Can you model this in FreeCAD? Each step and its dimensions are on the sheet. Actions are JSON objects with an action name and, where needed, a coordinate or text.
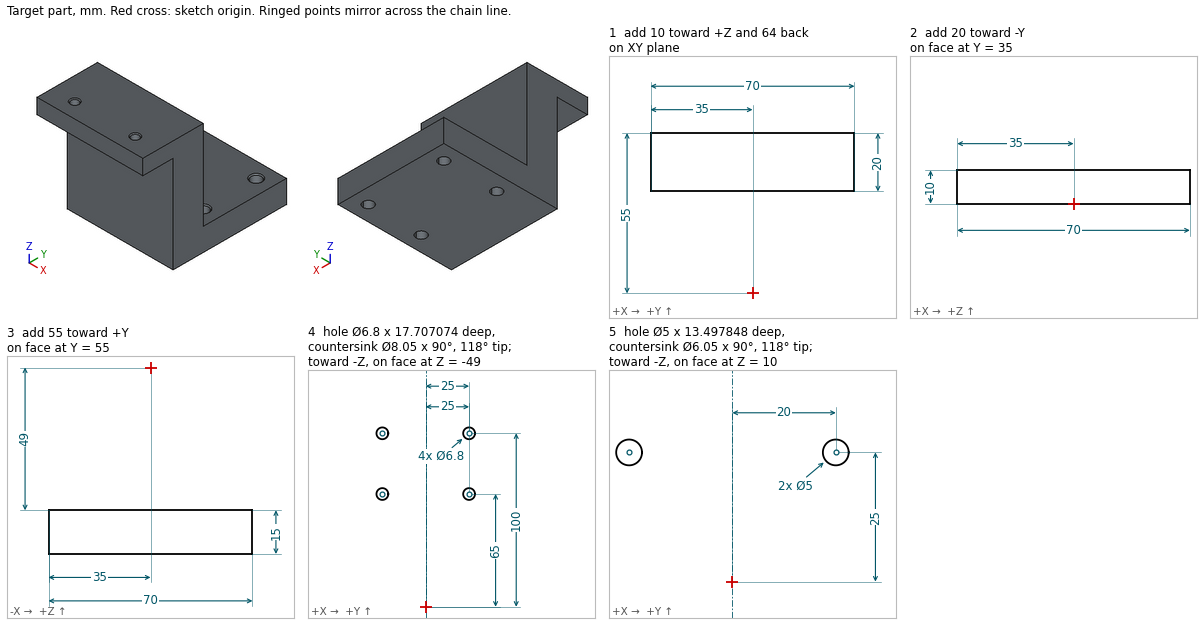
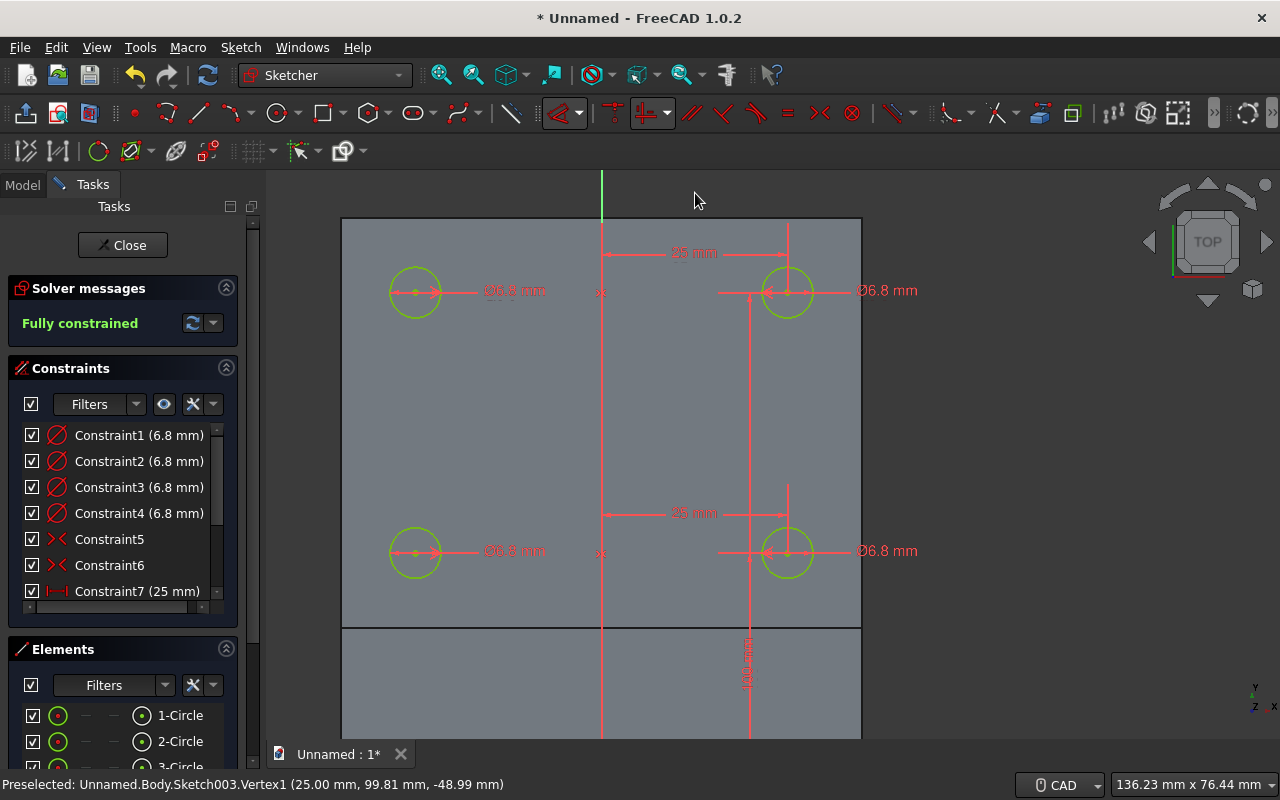
{"action": "left_click", "coordinate": [123, 245]}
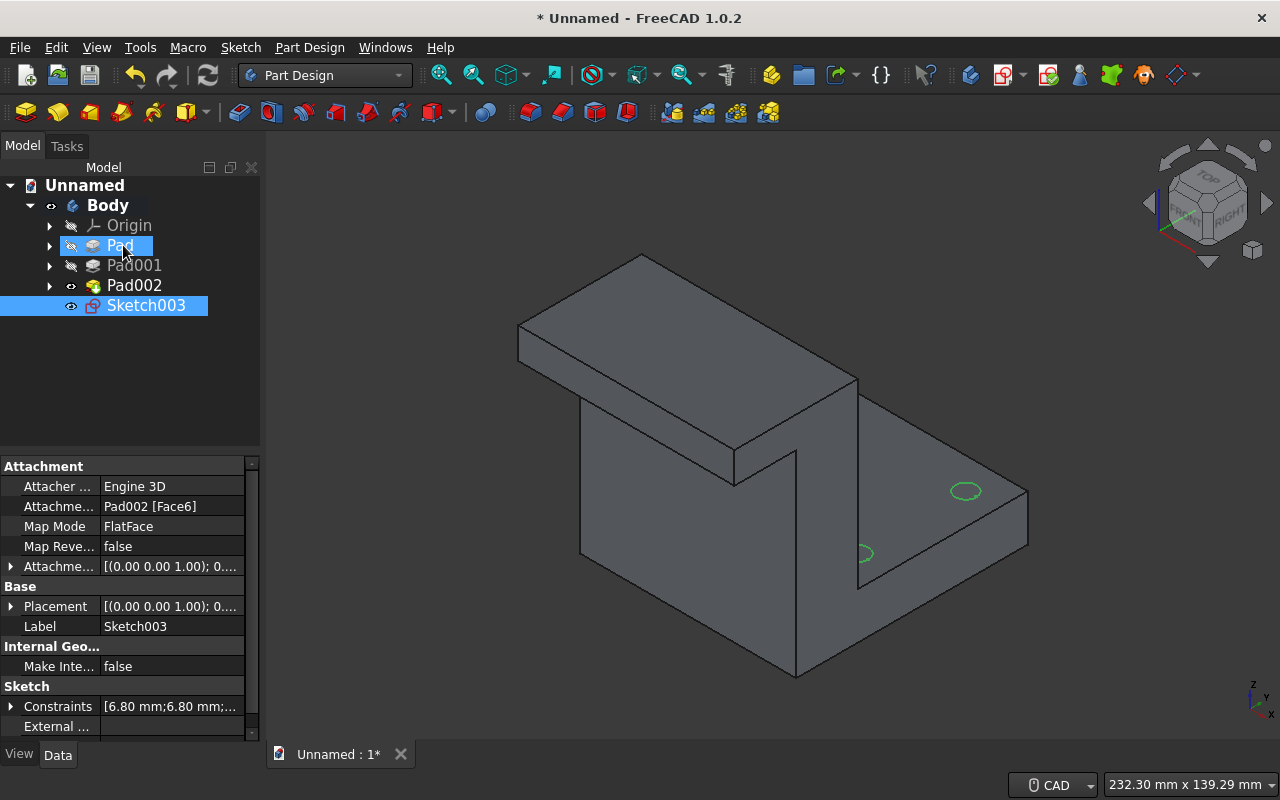
{"action": "left_click", "coordinate": [272, 112]}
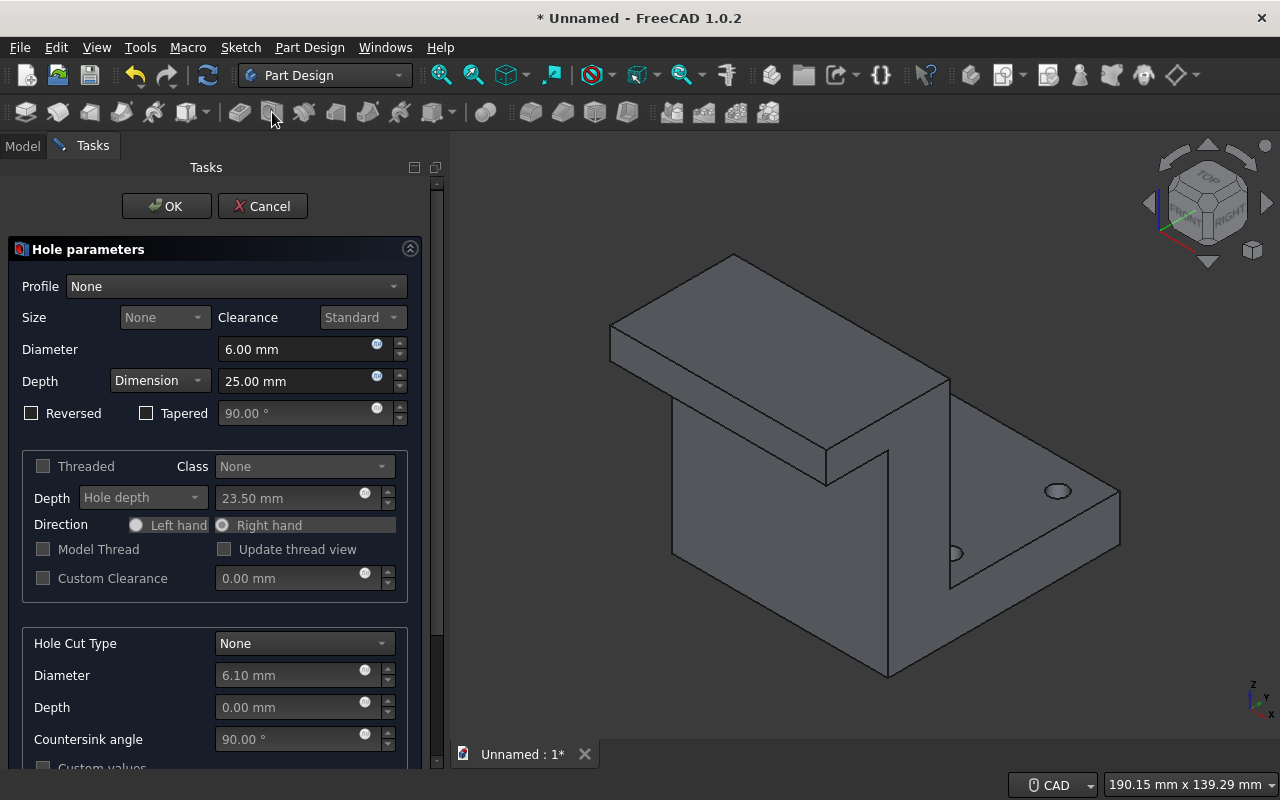
{"action": "triple_click", "coordinate": [305, 349]}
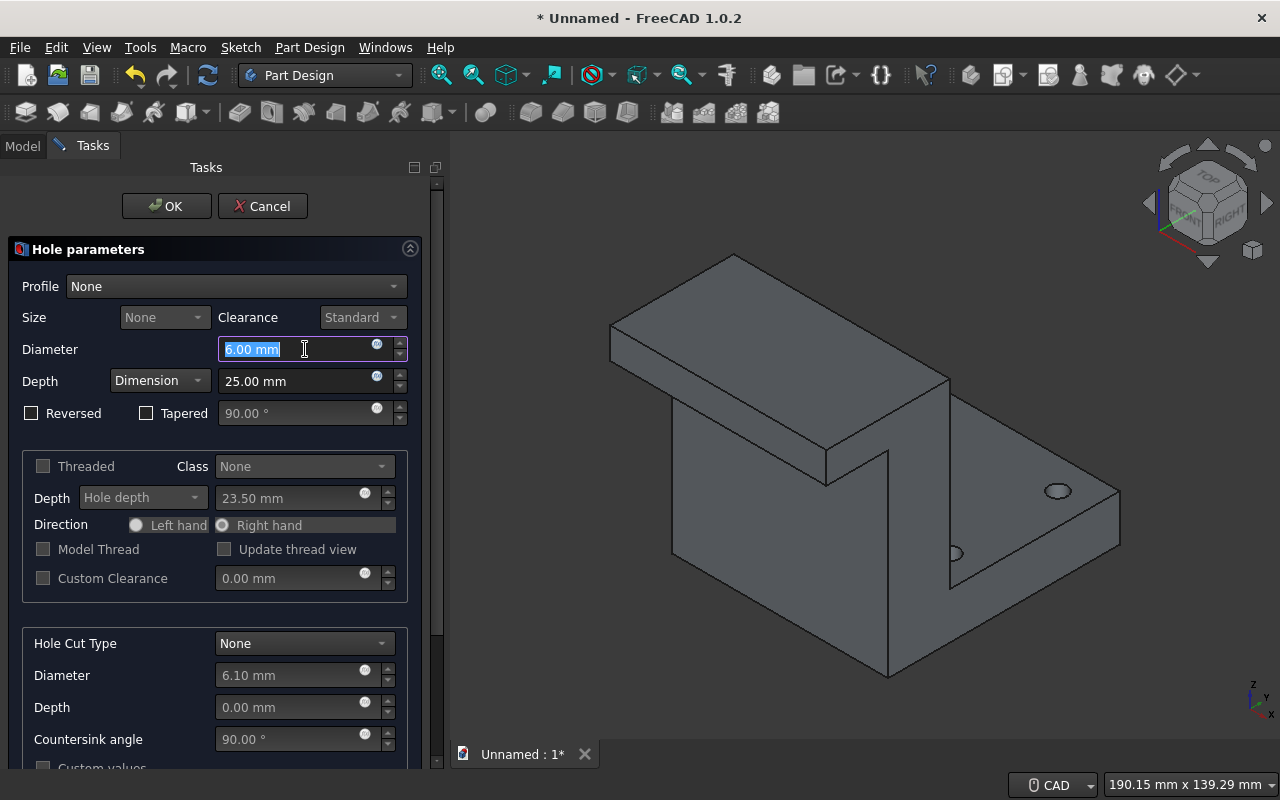
{"action": "type", "text": "6.8"}
{"action": "key", "text": "Tab"}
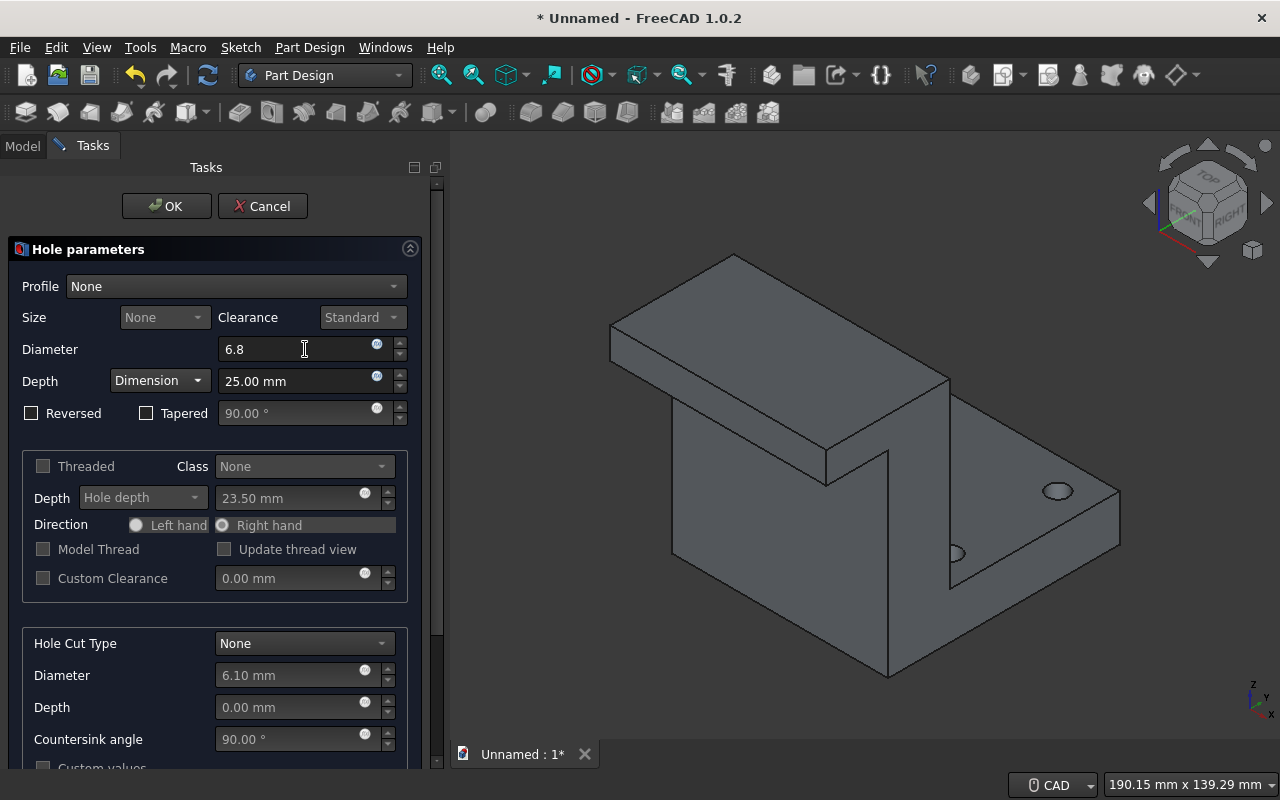
{"action": "triple_click", "coordinate": [305, 381]}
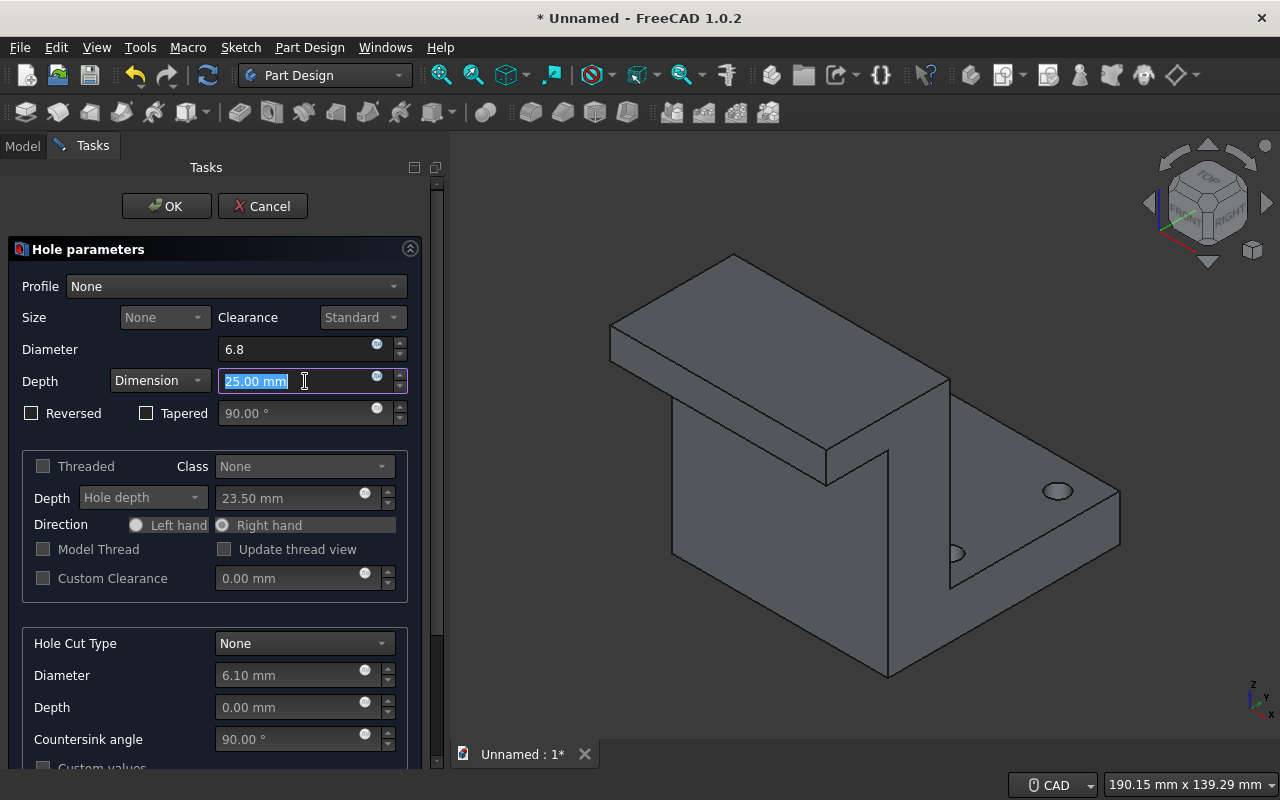
{"action": "type", "text": "17.707074"}
{"action": "key", "text": "Tab"}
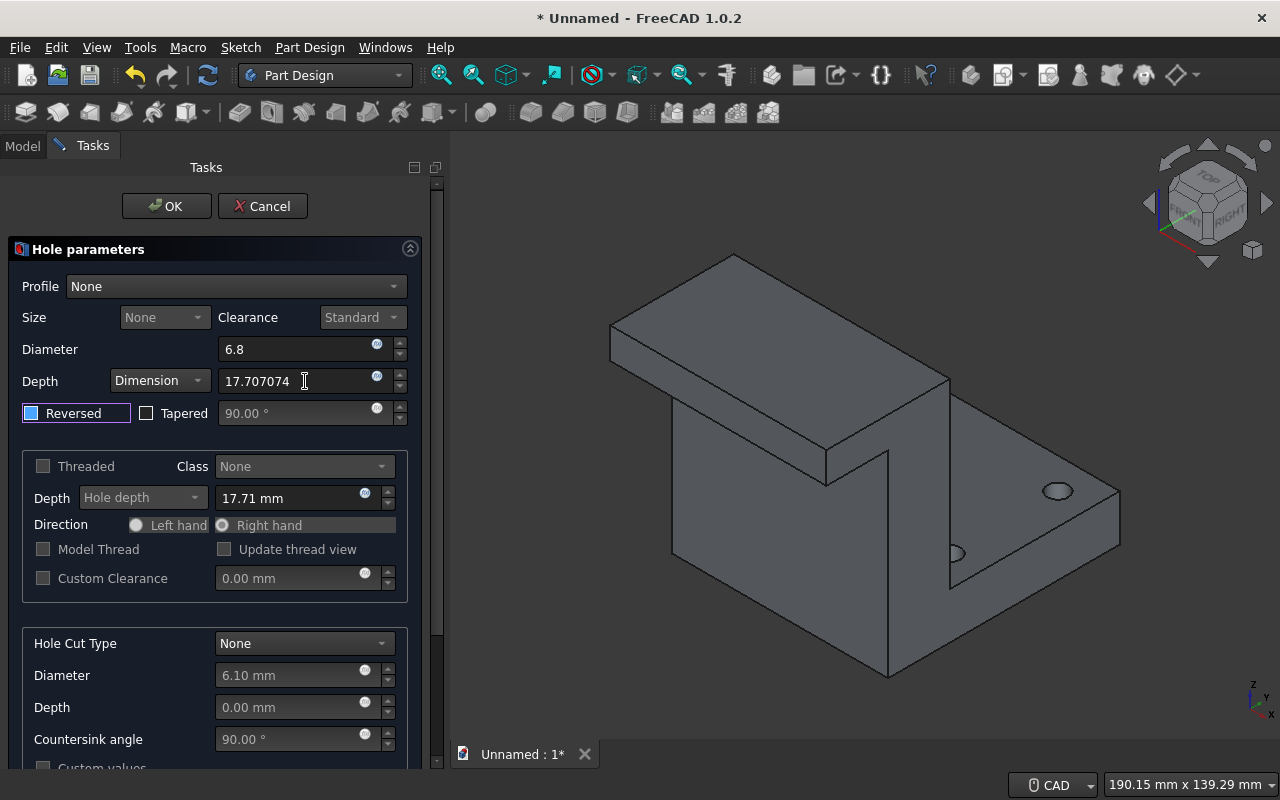
{"action": "left_click", "coordinate": [306, 644]}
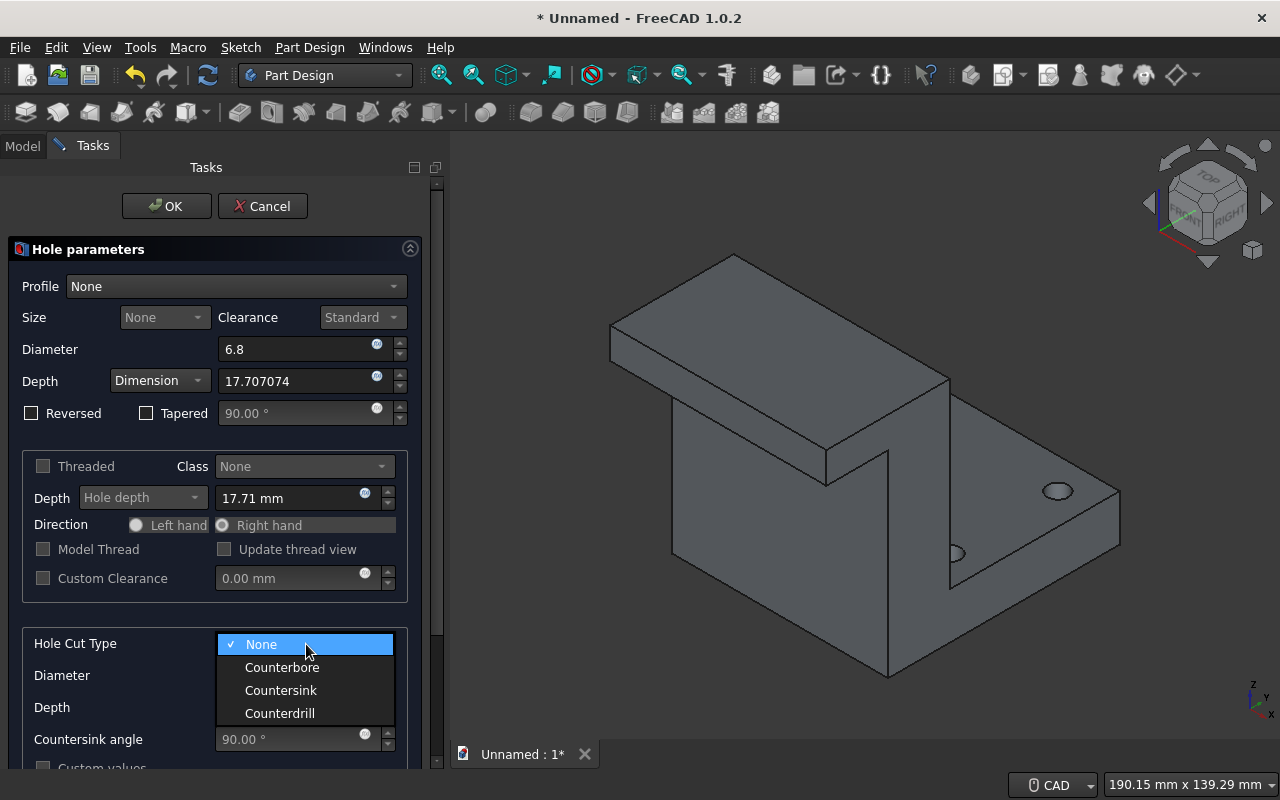
{"action": "left_click", "coordinate": [304, 690]}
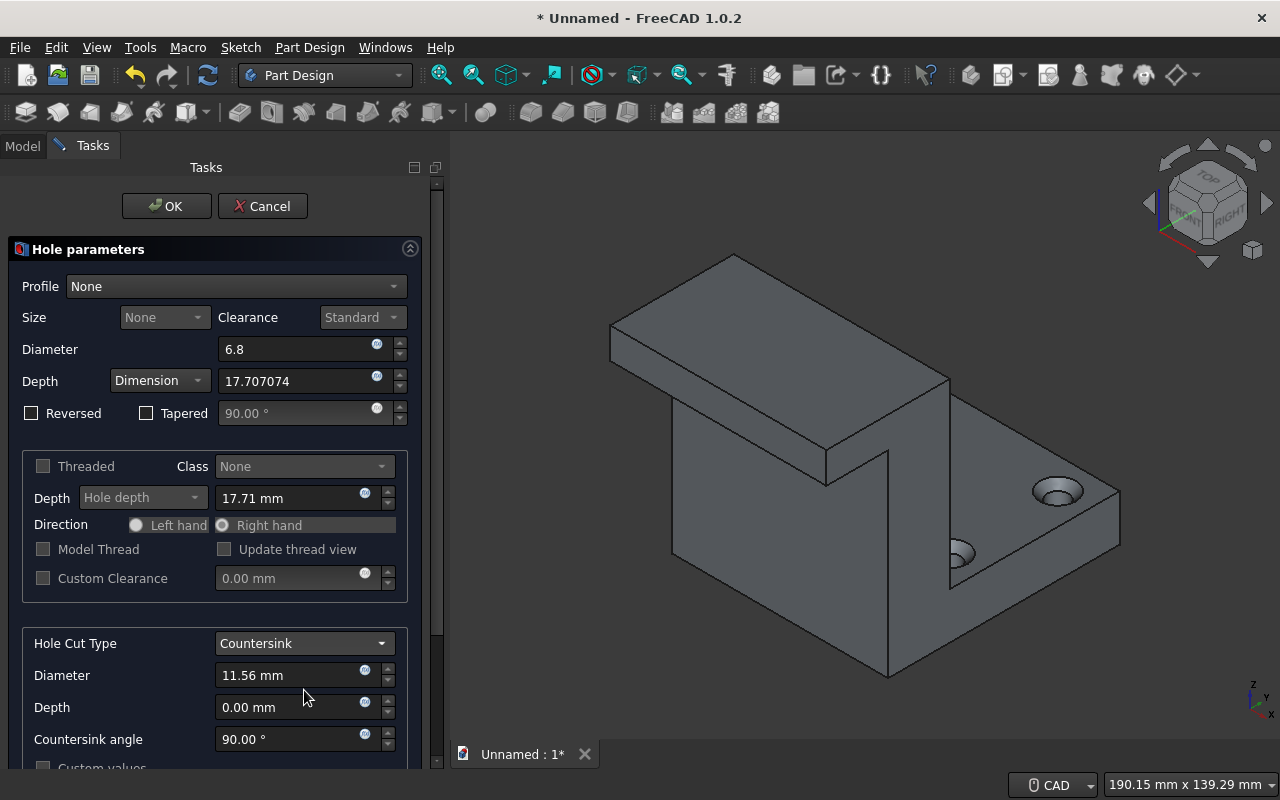
{"action": "triple_click", "coordinate": [298, 675]}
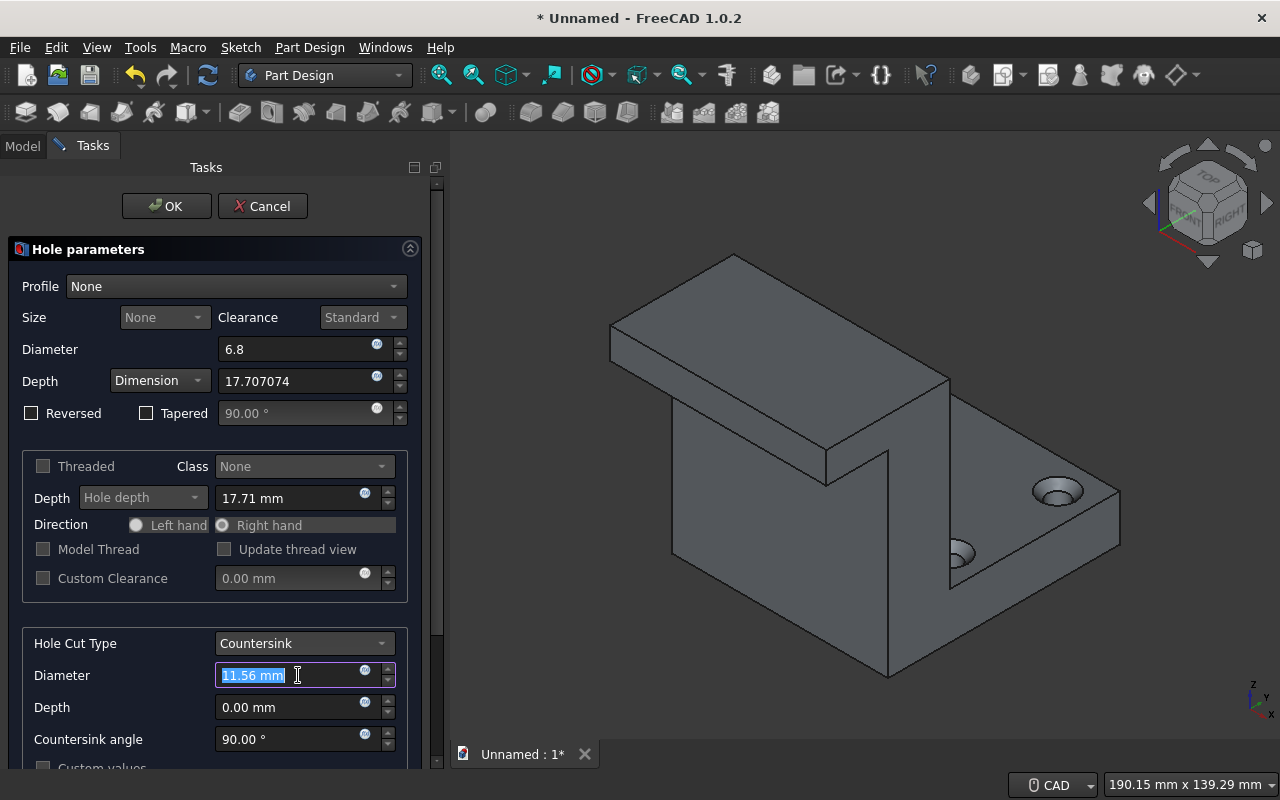
{"action": "type", "text": "8.05"}
{"action": "key", "text": "Tab"}